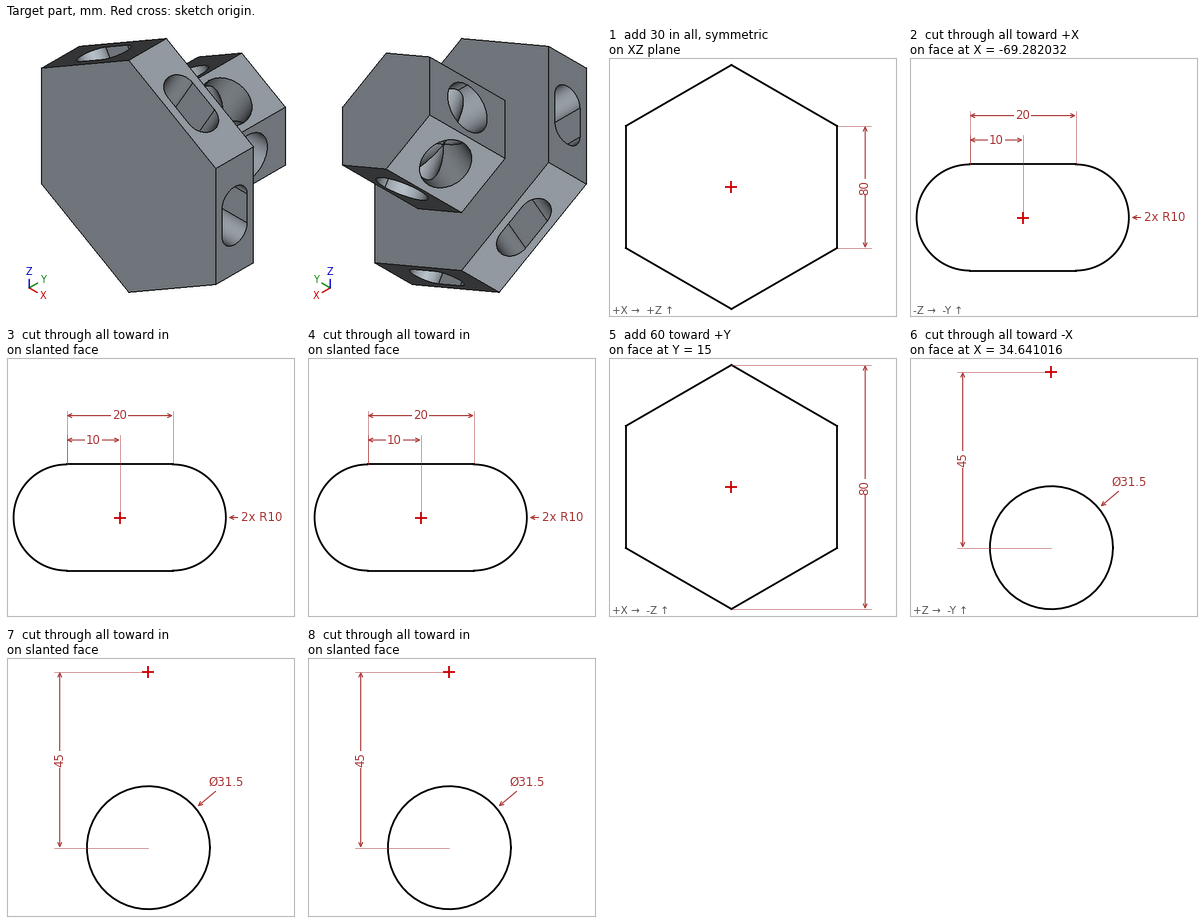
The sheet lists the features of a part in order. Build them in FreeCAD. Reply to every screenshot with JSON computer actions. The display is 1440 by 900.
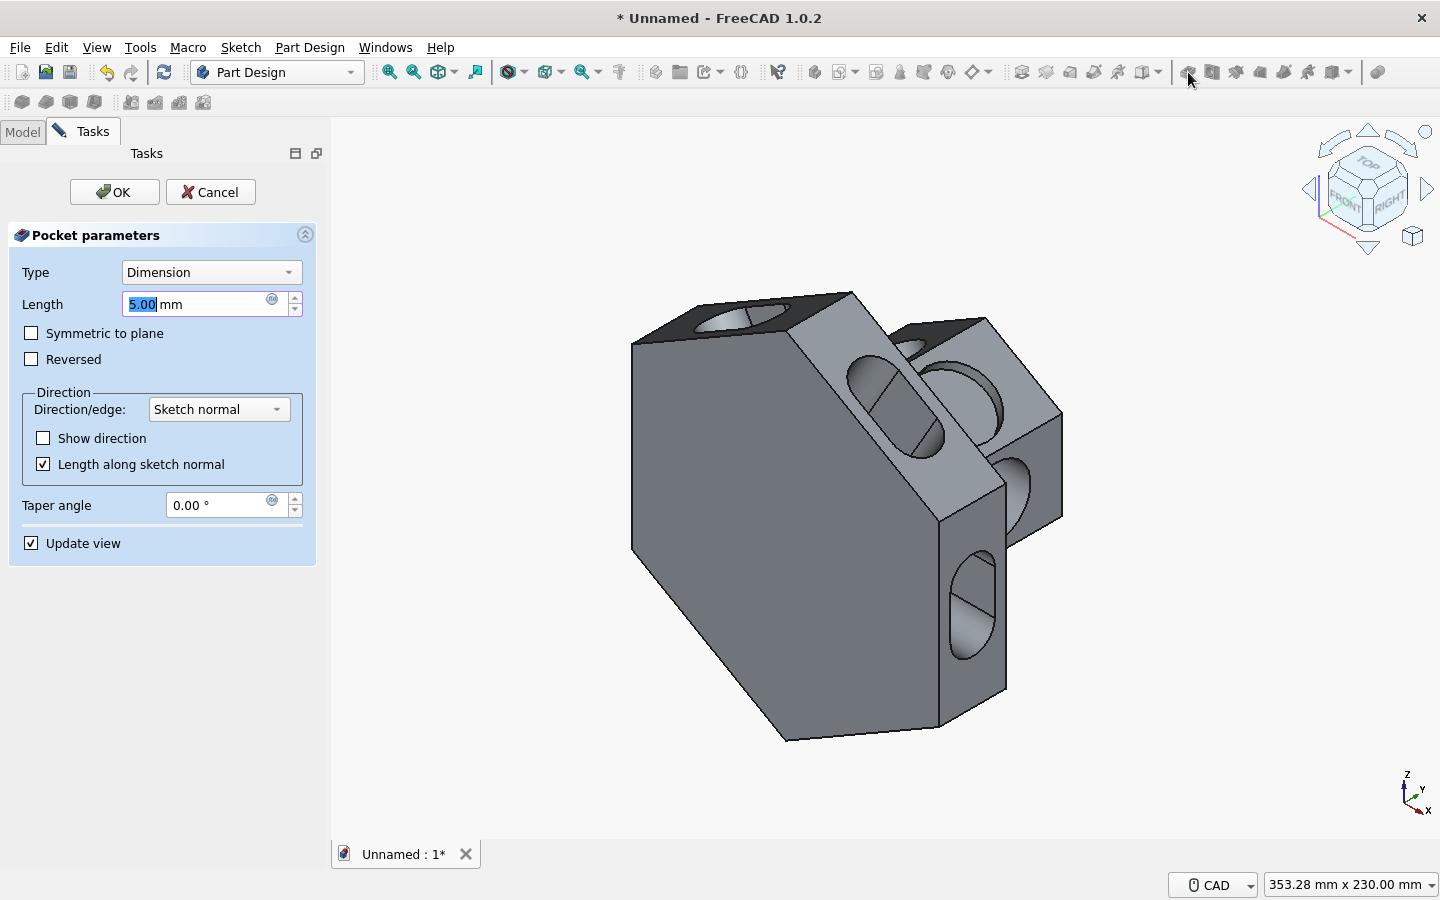
{"action": "left_click", "coordinate": [212, 272]}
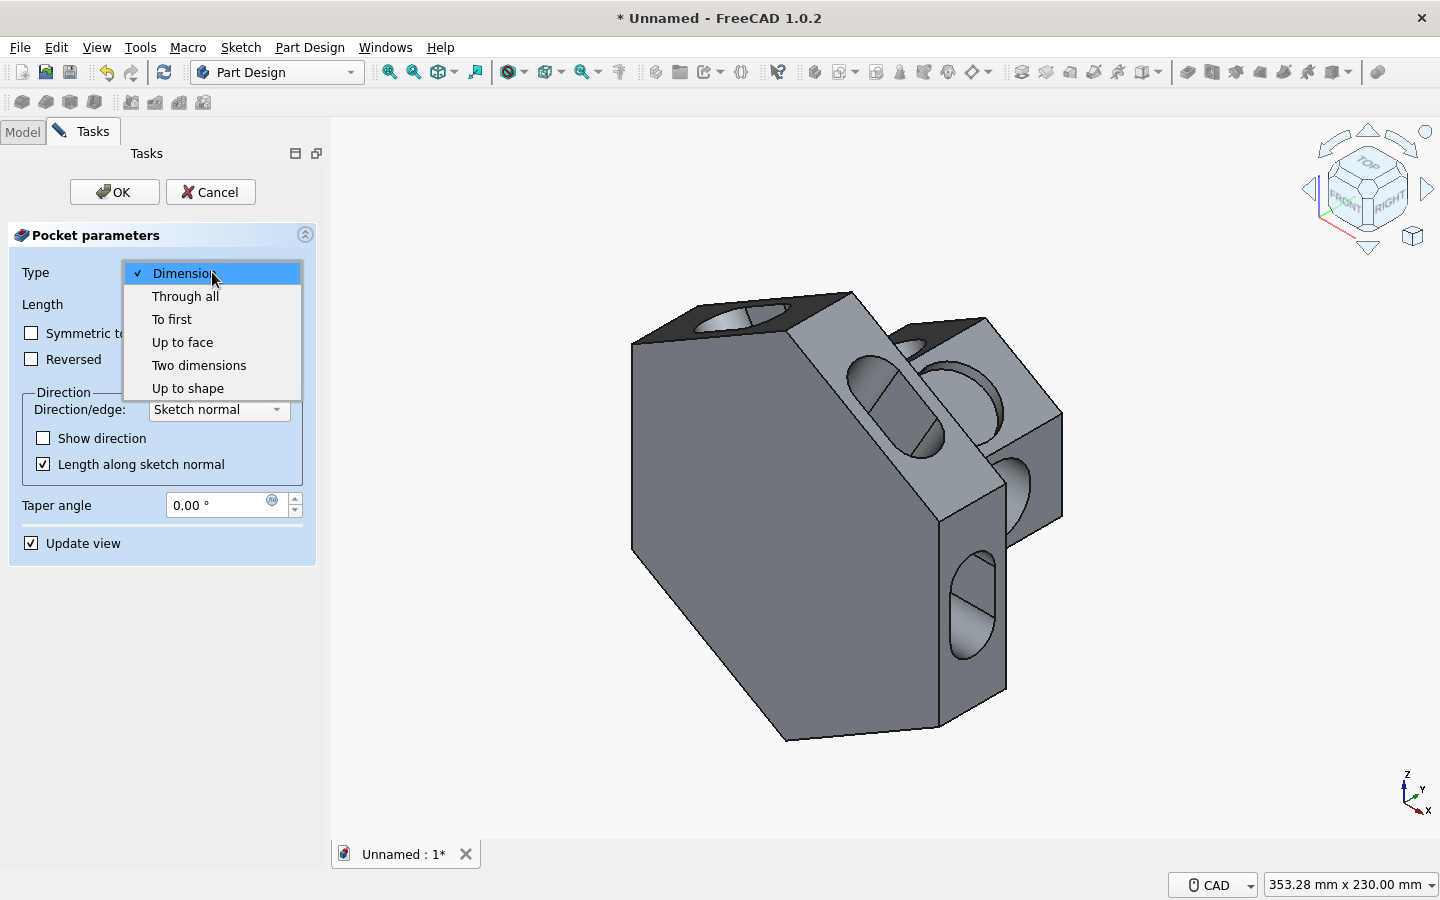
{"action": "left_click", "coordinate": [212, 296]}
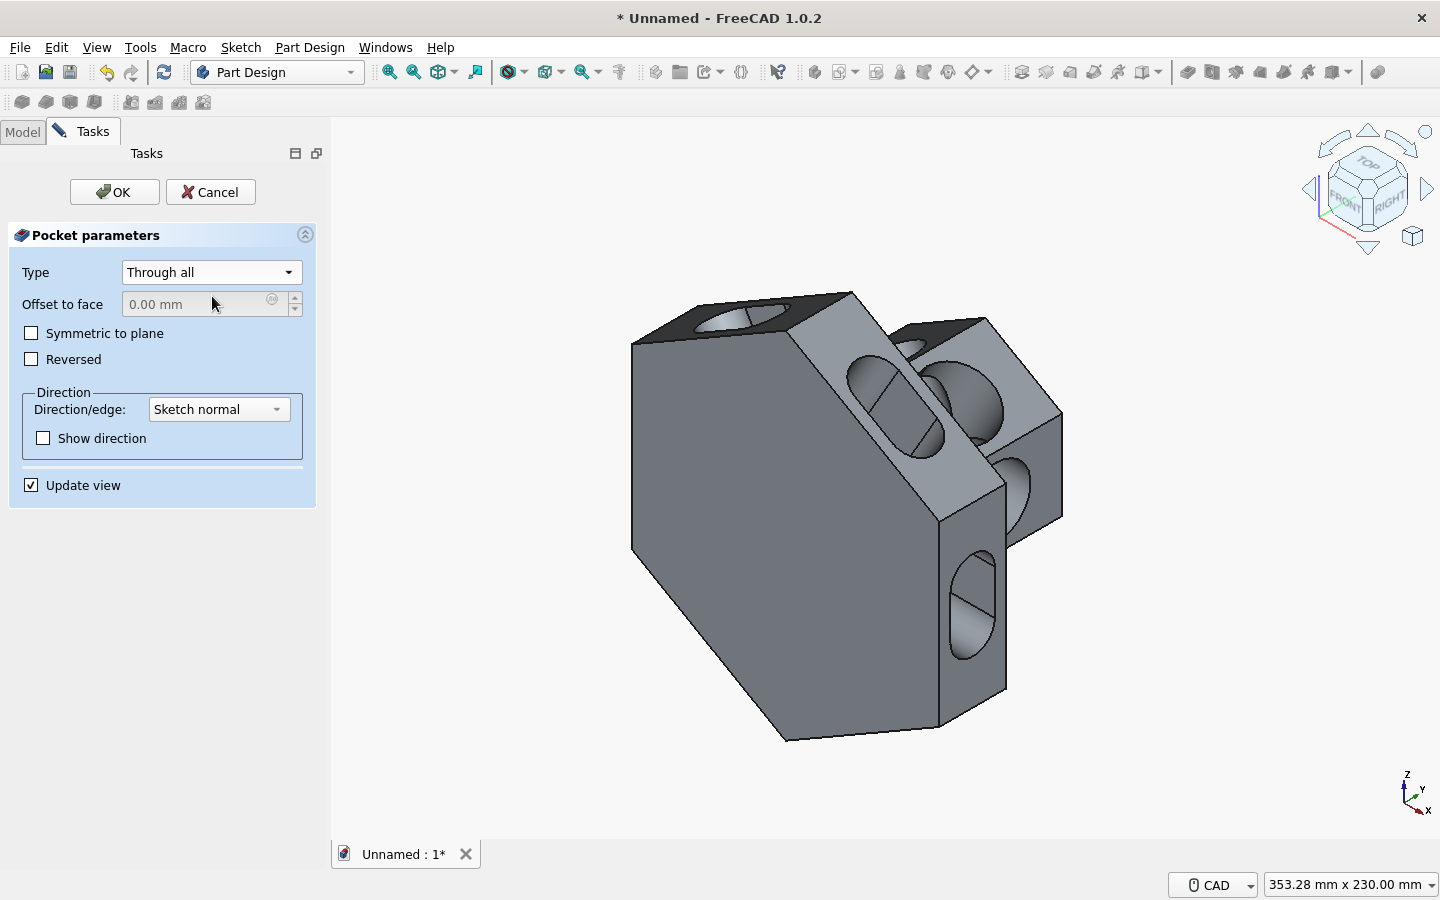
{"action": "left_click", "coordinate": [115, 192]}